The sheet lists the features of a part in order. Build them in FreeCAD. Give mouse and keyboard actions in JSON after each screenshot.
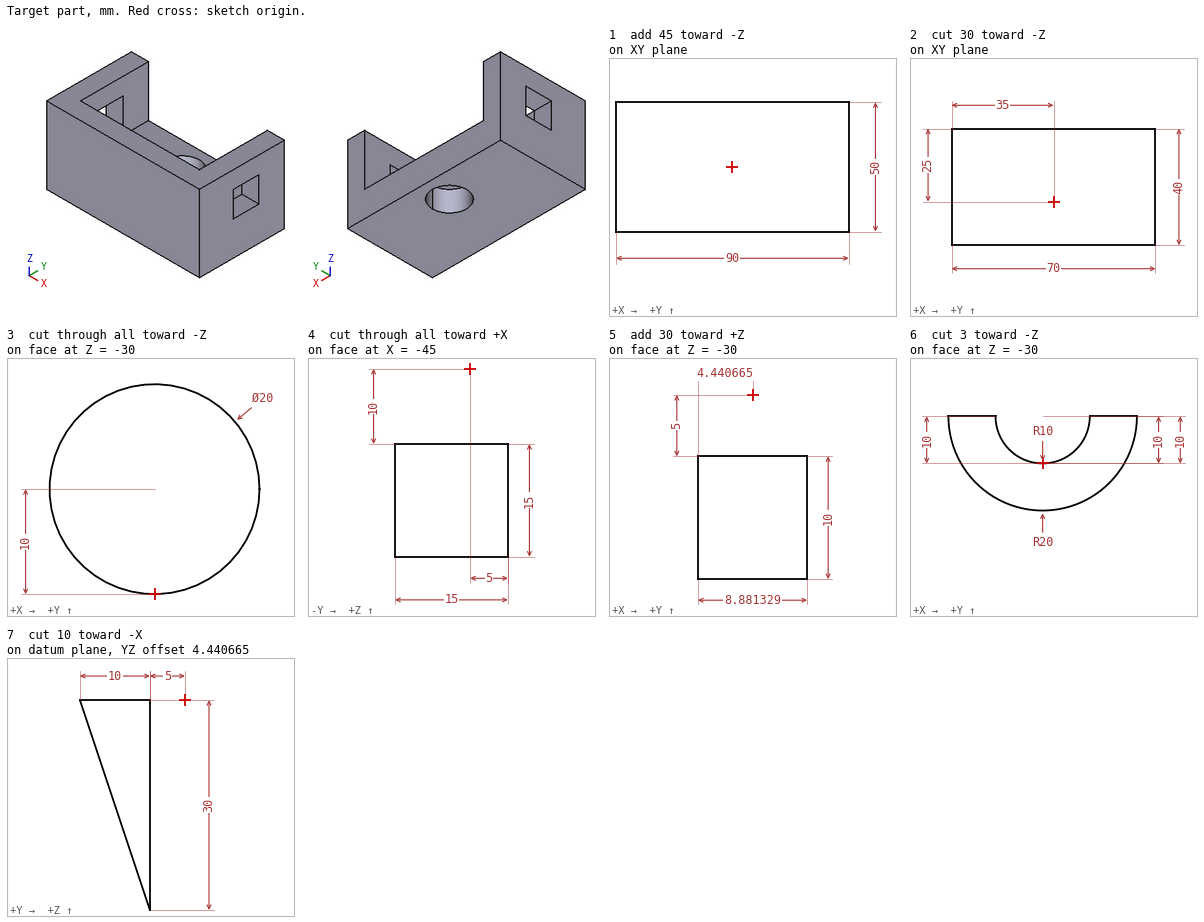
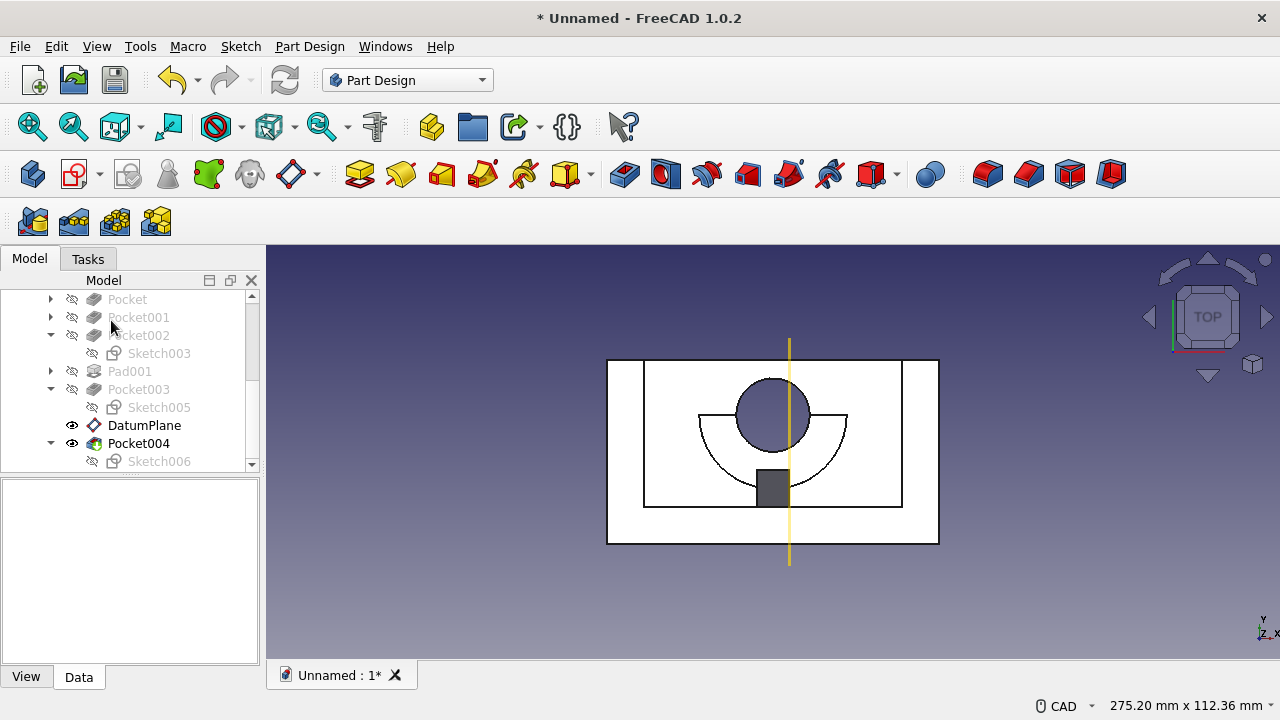
{"action": "left_click", "coordinate": [117, 425]}
{"action": "key", "text": "space"}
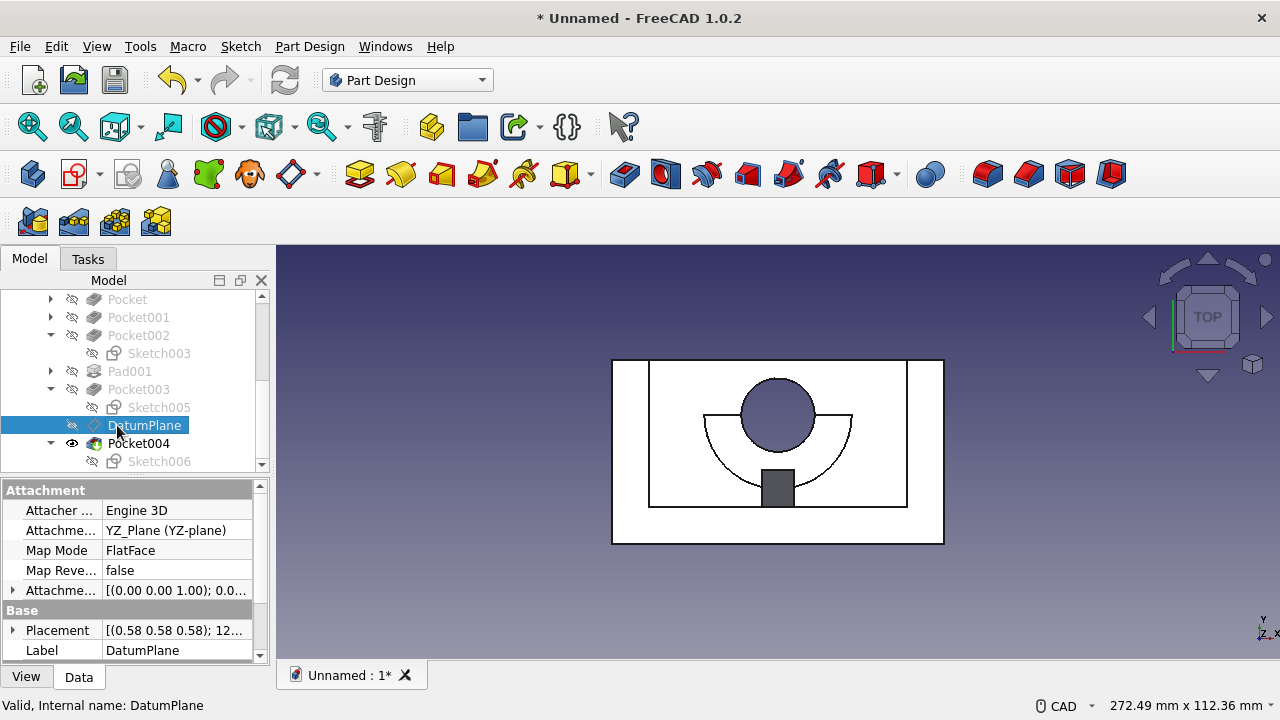
{"action": "key", "text": "0"}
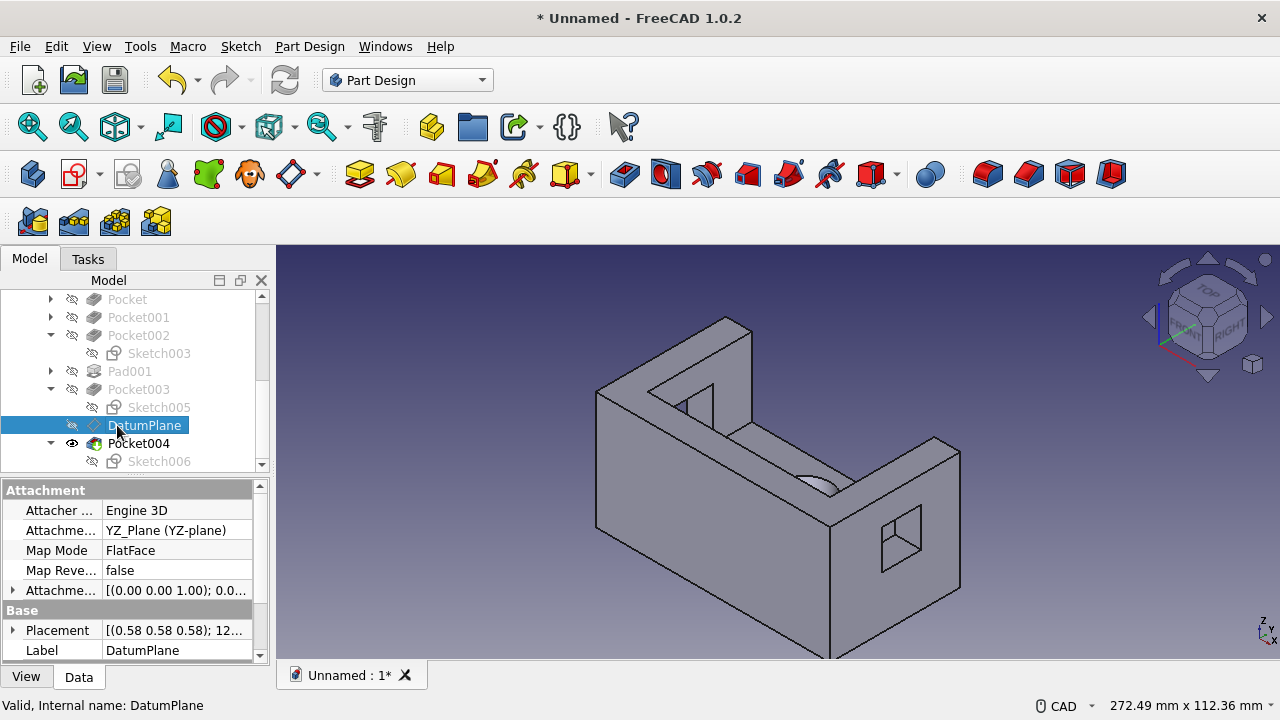
{"action": "key", "text": "v f"}